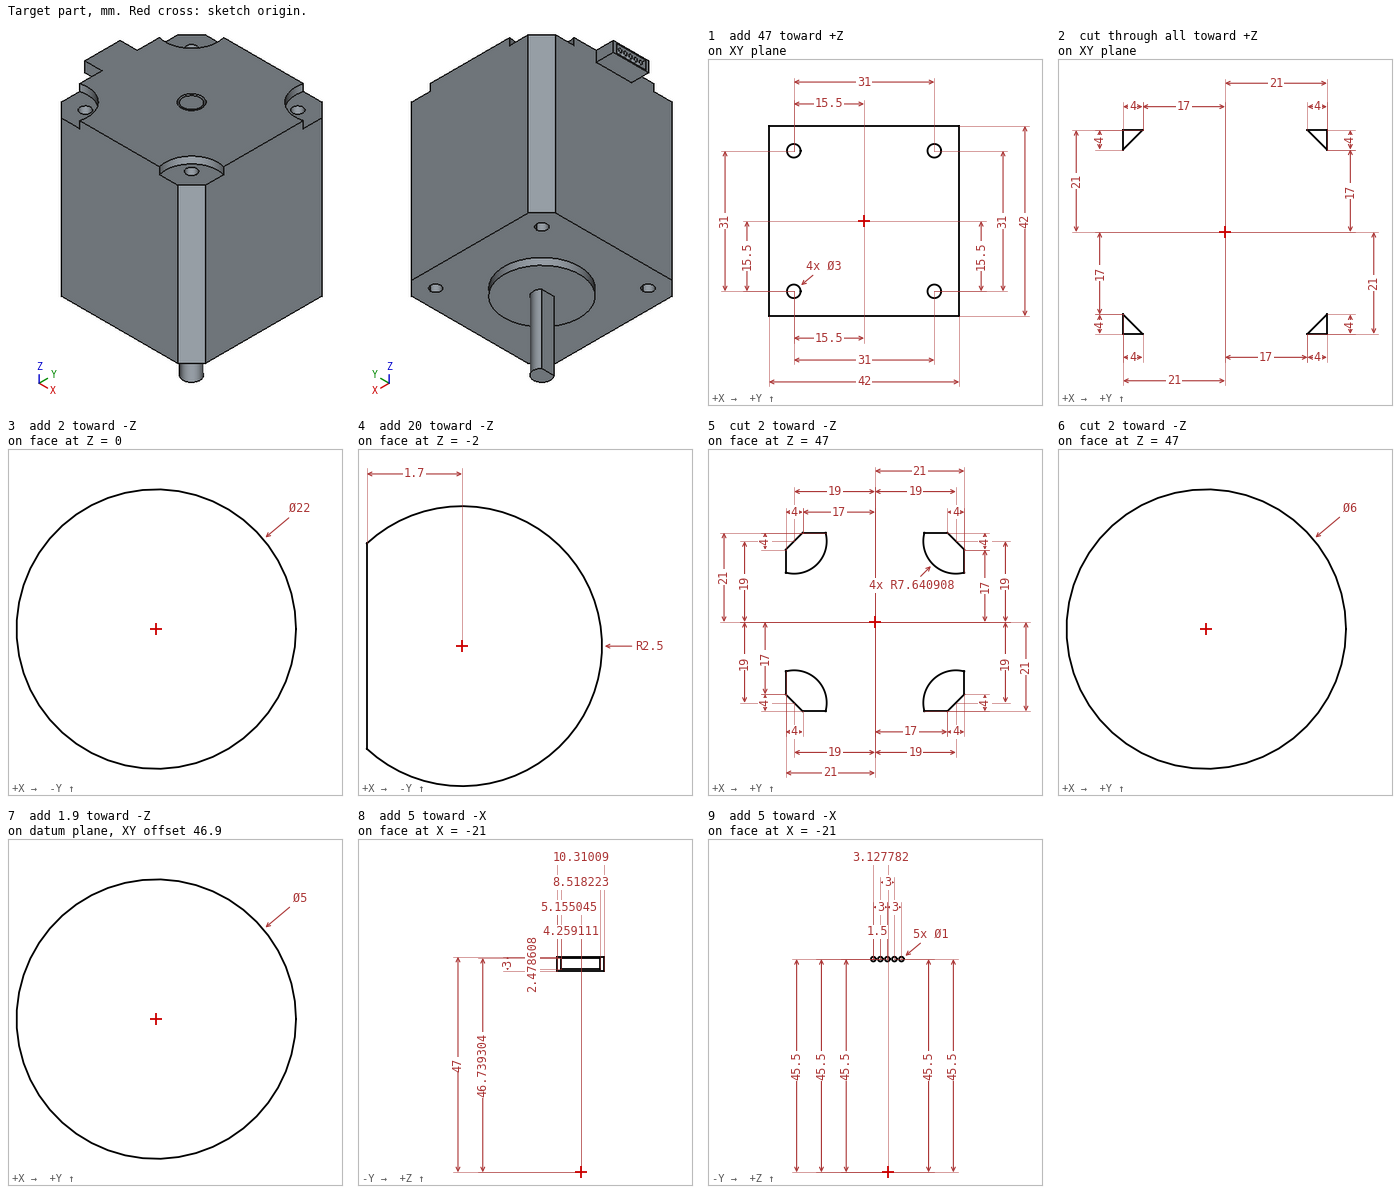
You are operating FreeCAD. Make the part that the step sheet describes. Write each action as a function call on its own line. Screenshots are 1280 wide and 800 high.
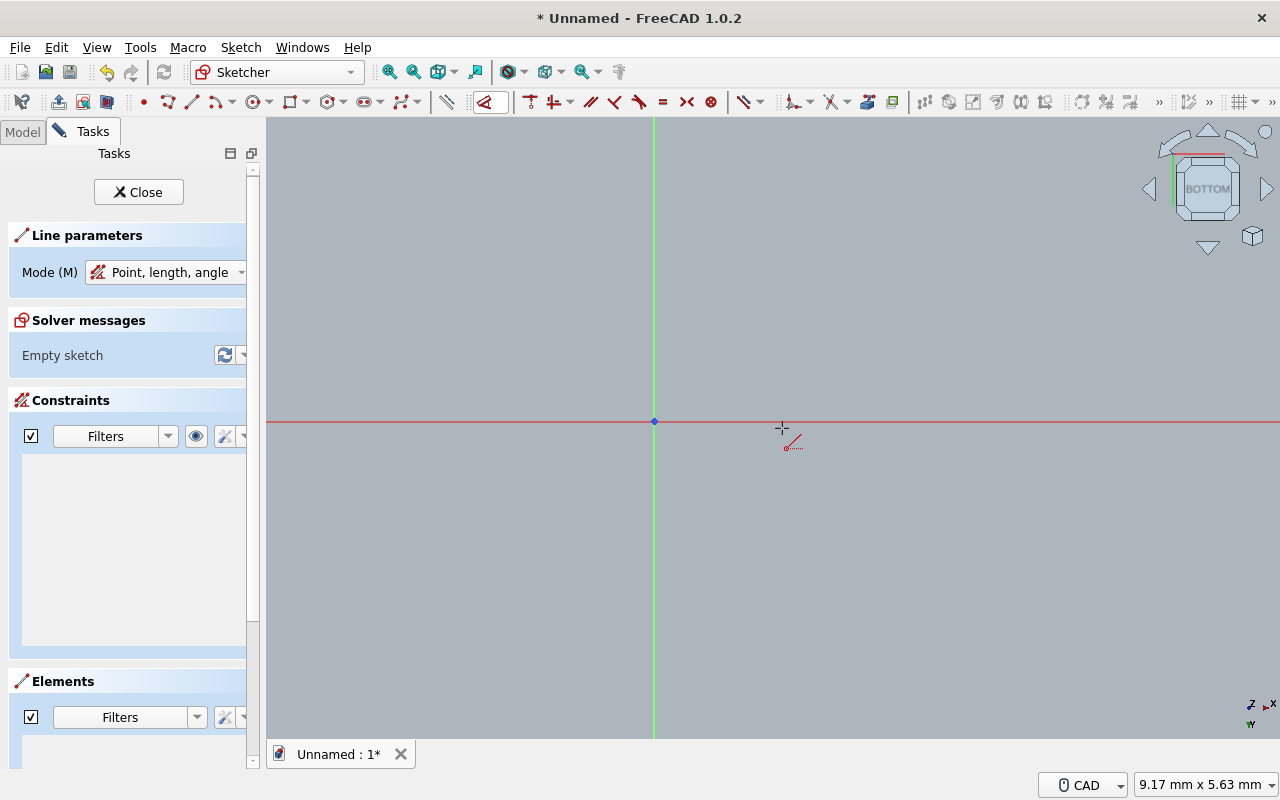
click(467, 219)
click(467, 624)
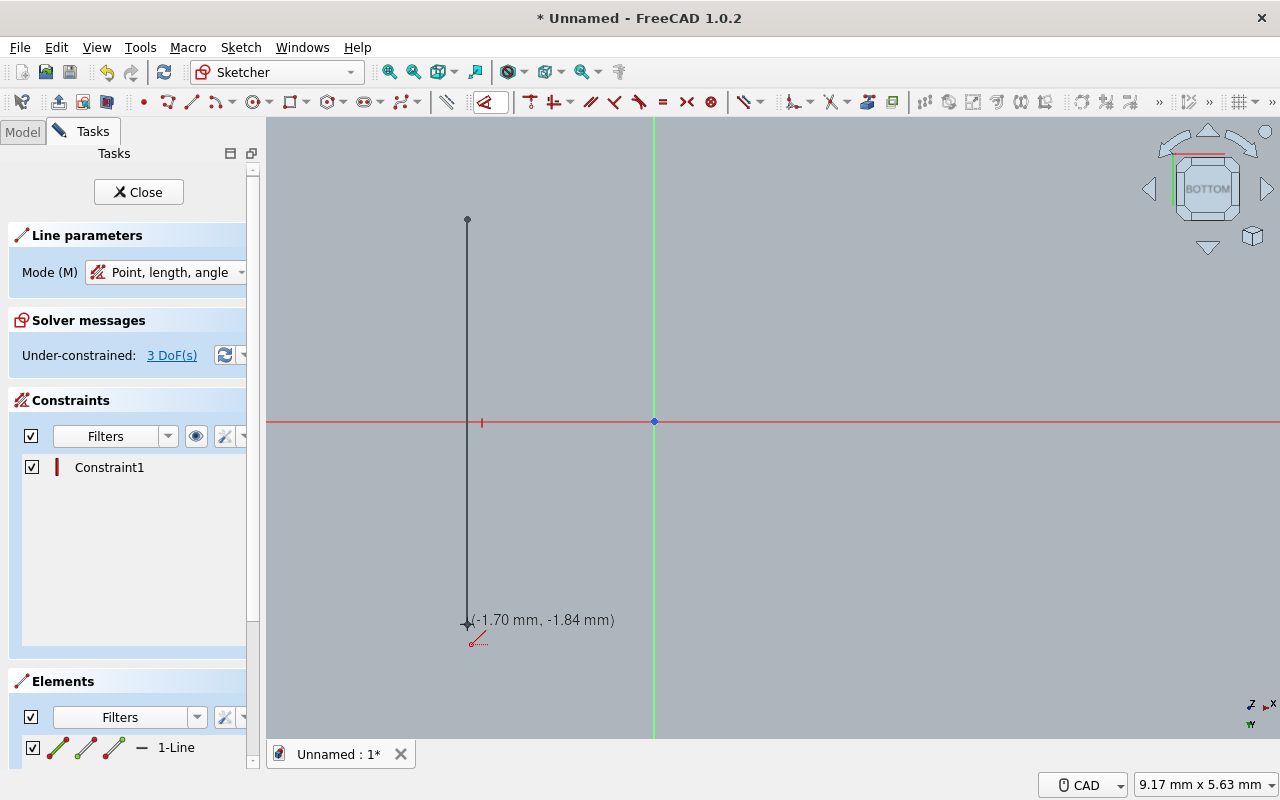
key(g)
key(3)
key(a)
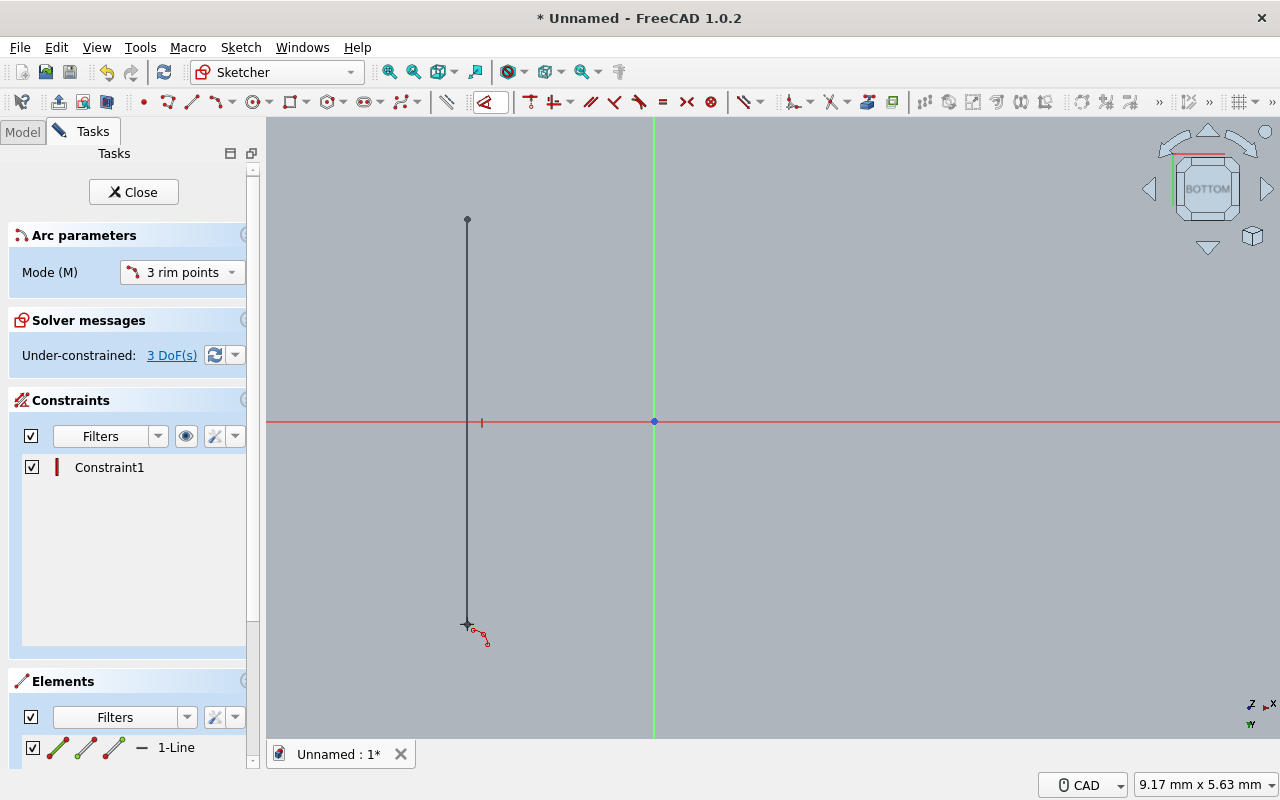
click(467, 625)
click(467, 220)
click(902, 545)
key(Escape)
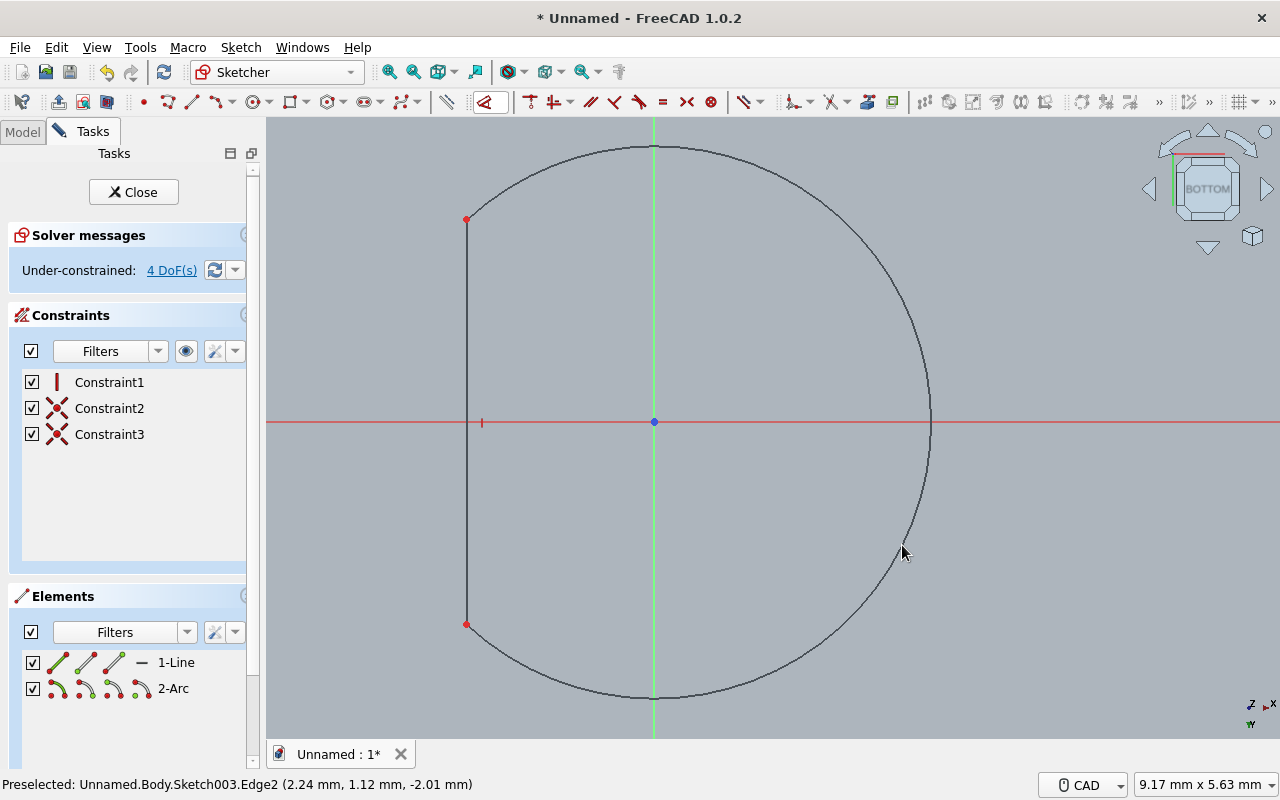
drag(644, 412, 665, 433)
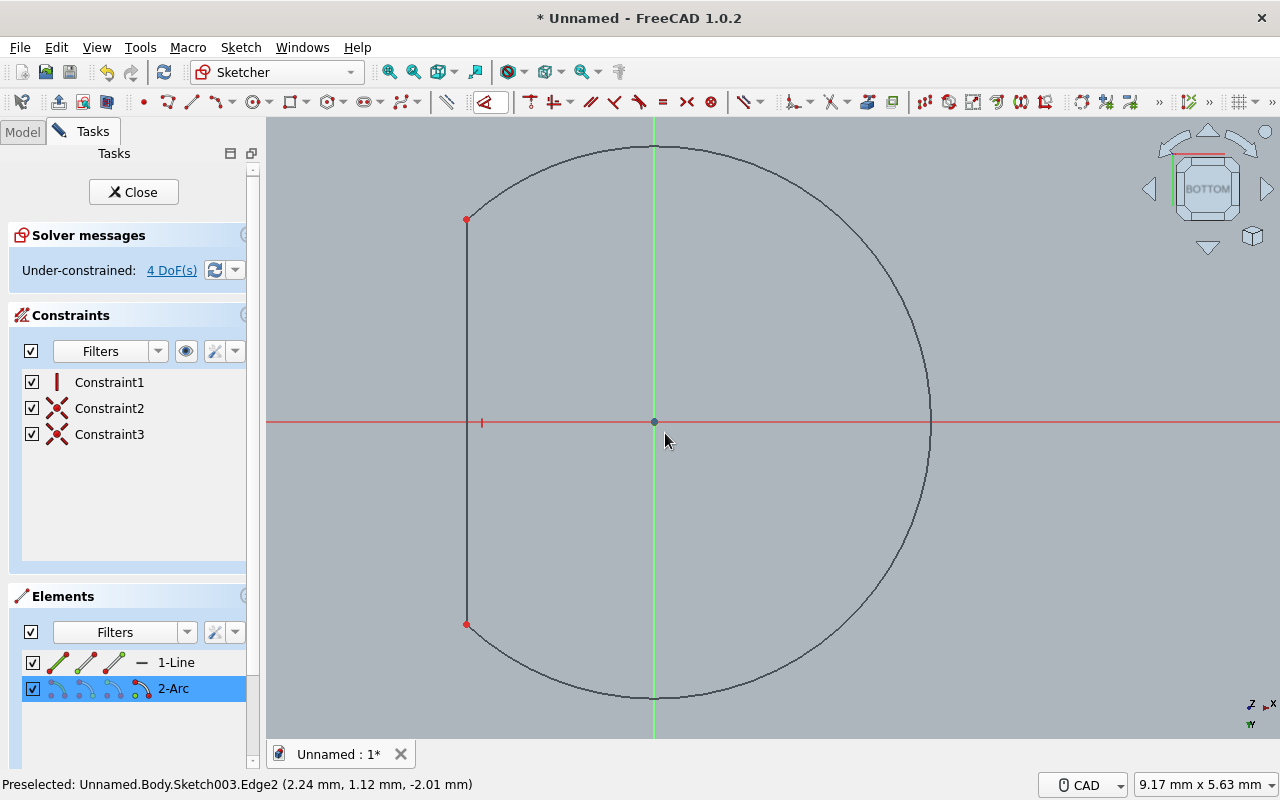
click(530, 102)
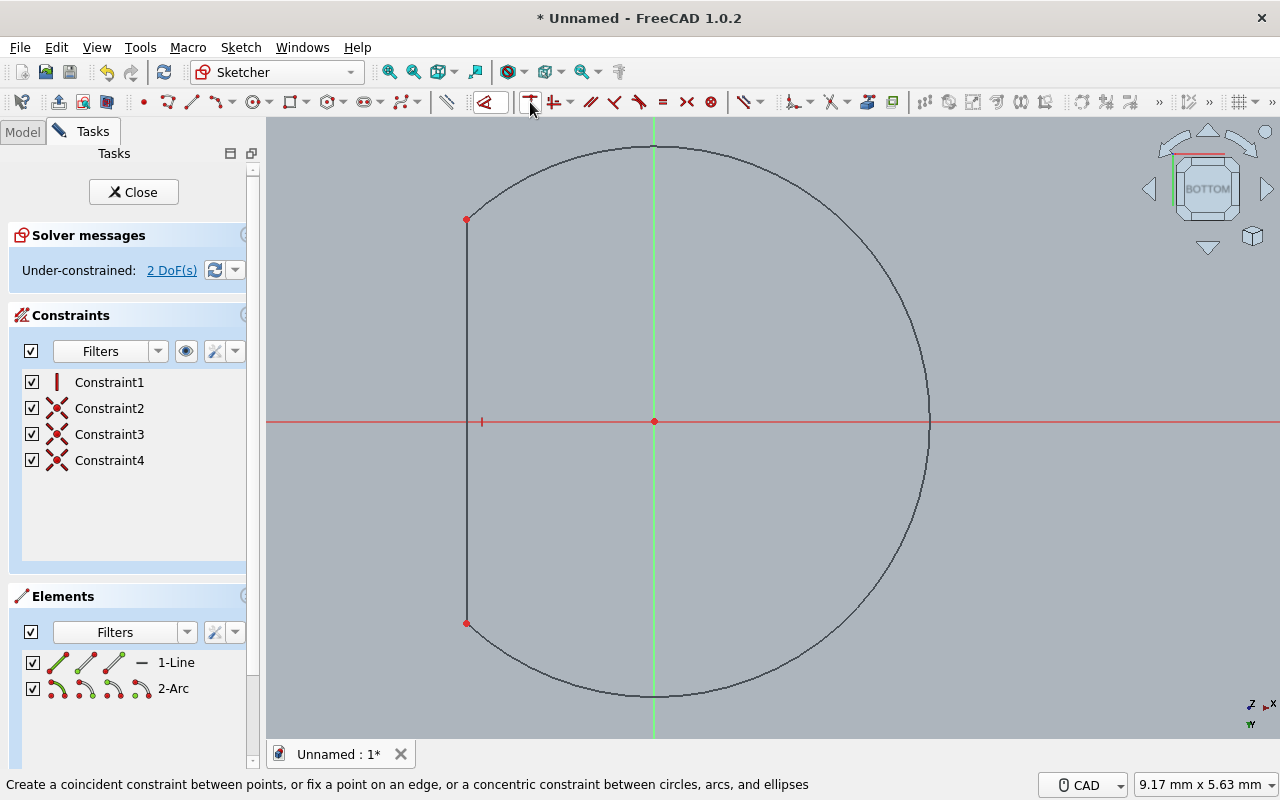
click(820, 642)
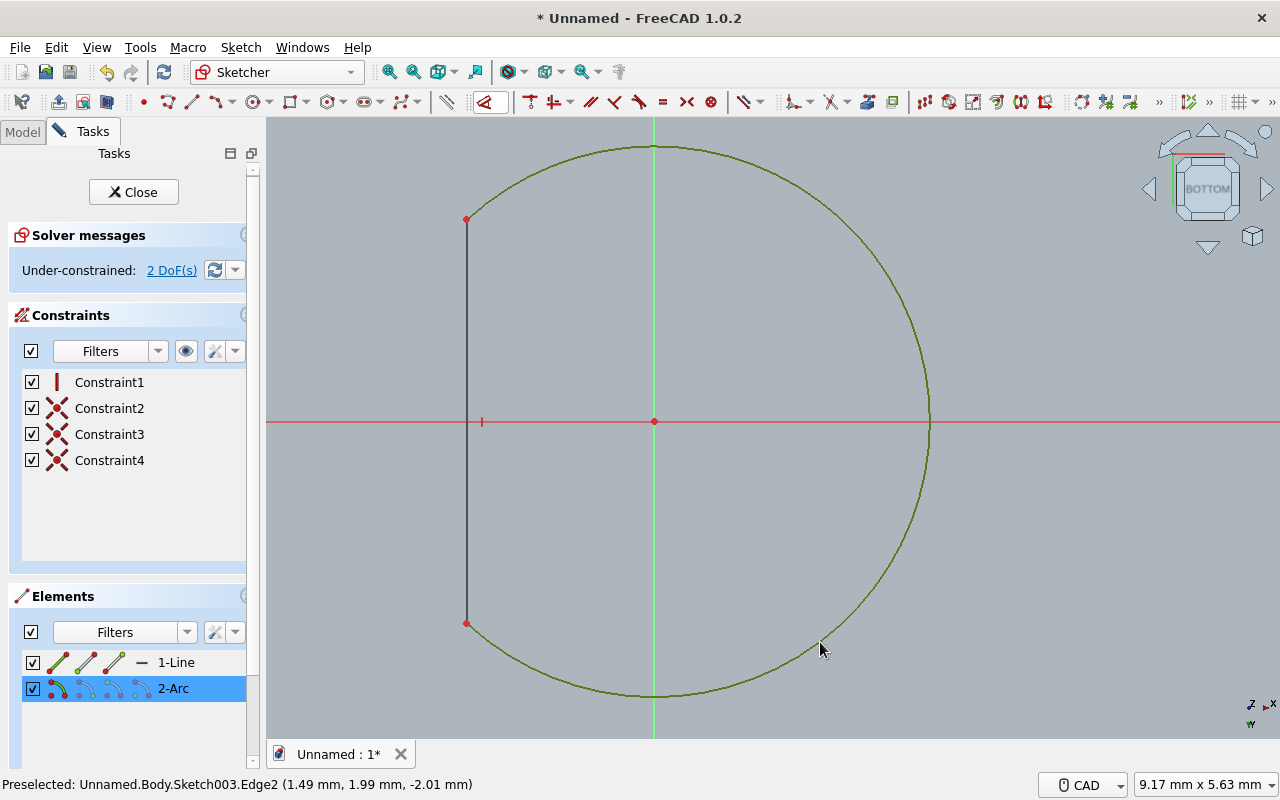
key(k)
key(r)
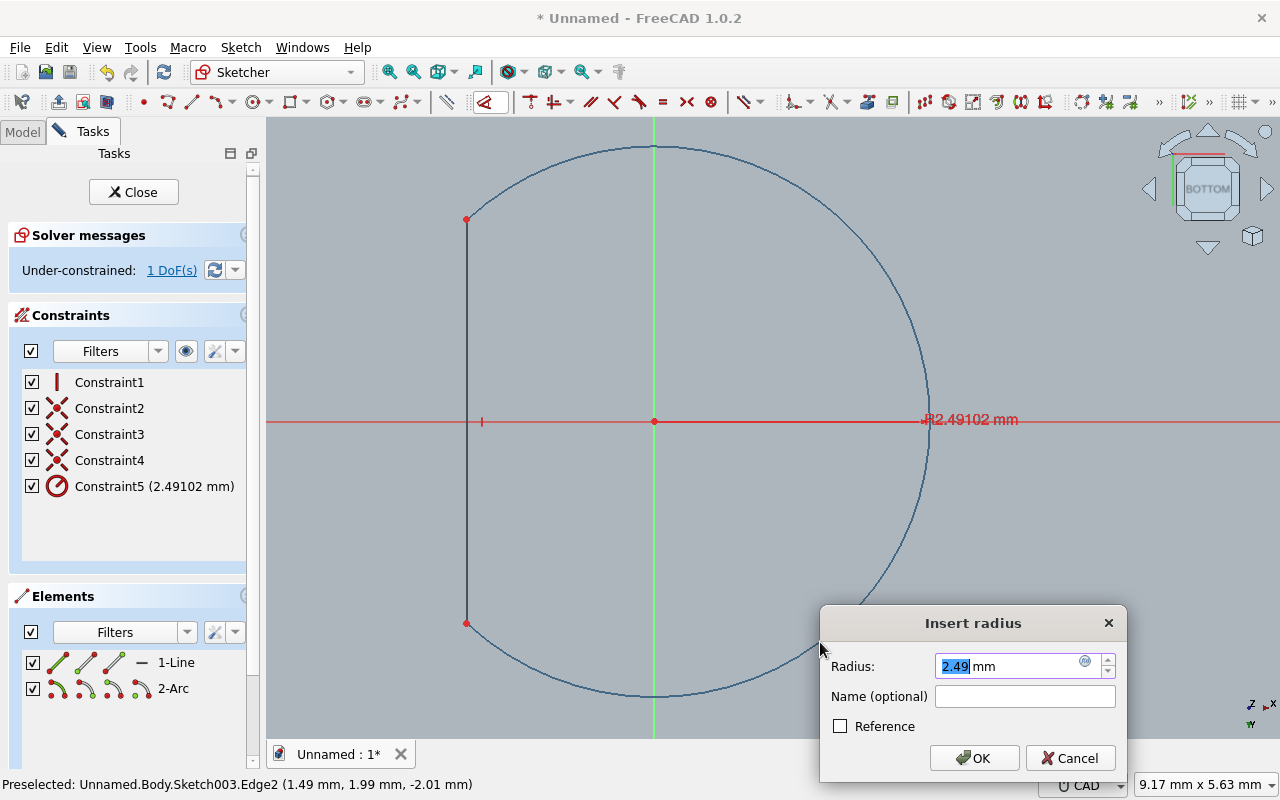
text(2.5)
key(Return)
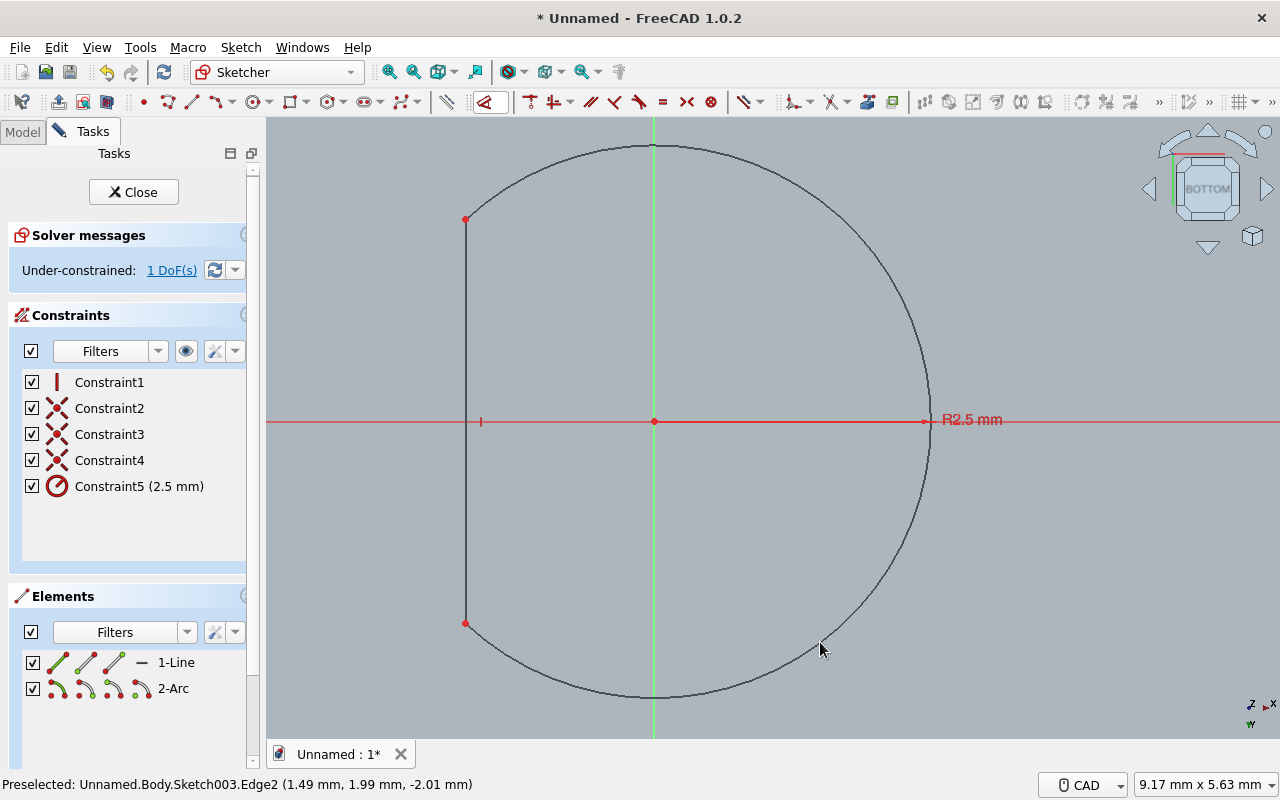
click(466, 220)